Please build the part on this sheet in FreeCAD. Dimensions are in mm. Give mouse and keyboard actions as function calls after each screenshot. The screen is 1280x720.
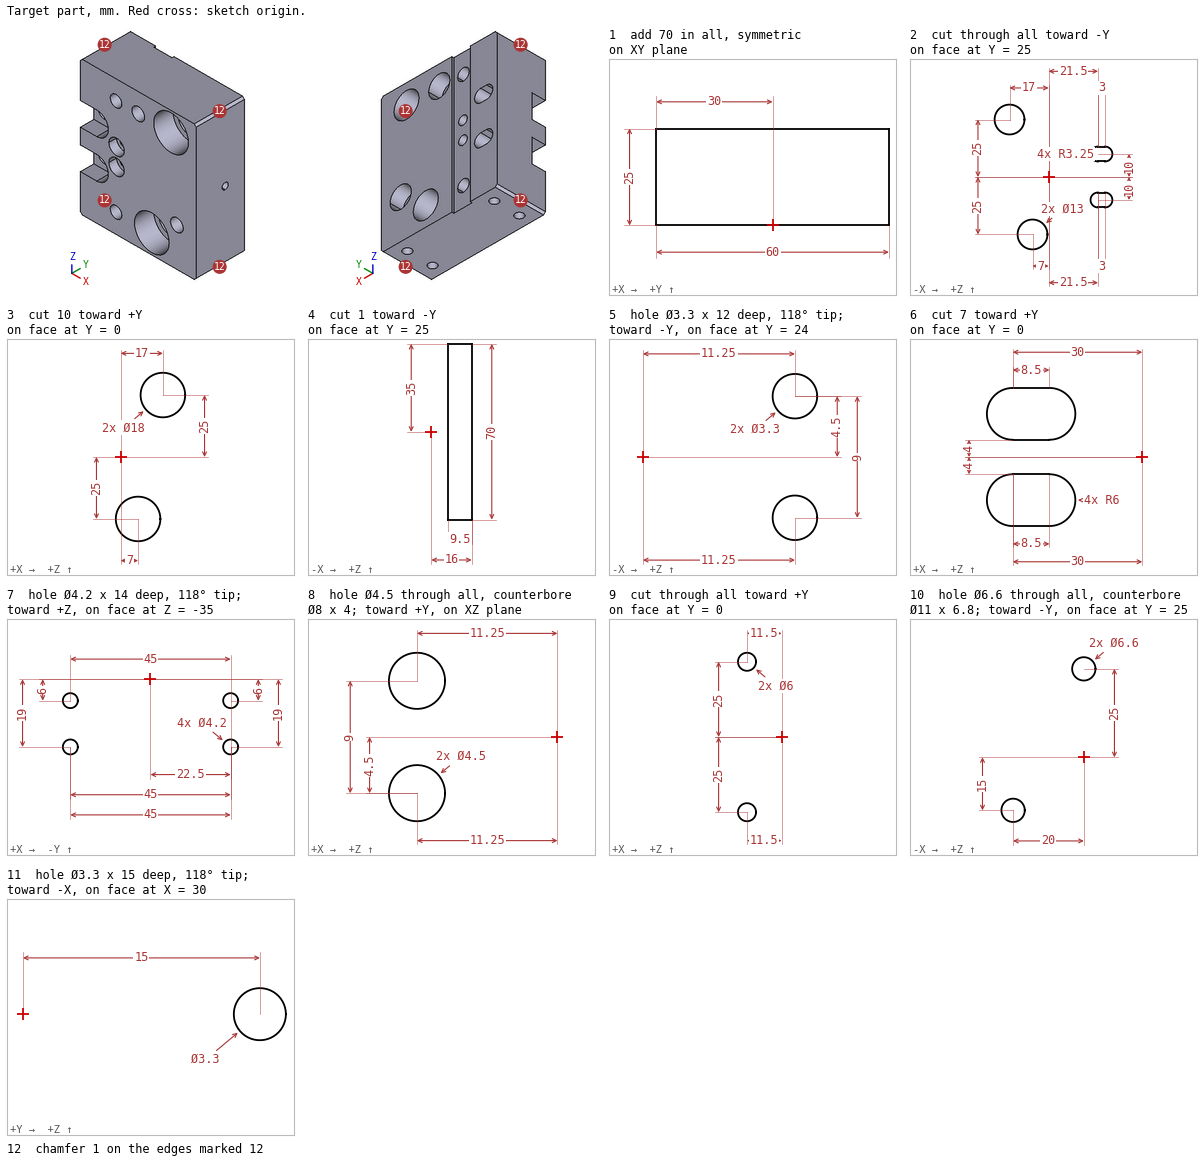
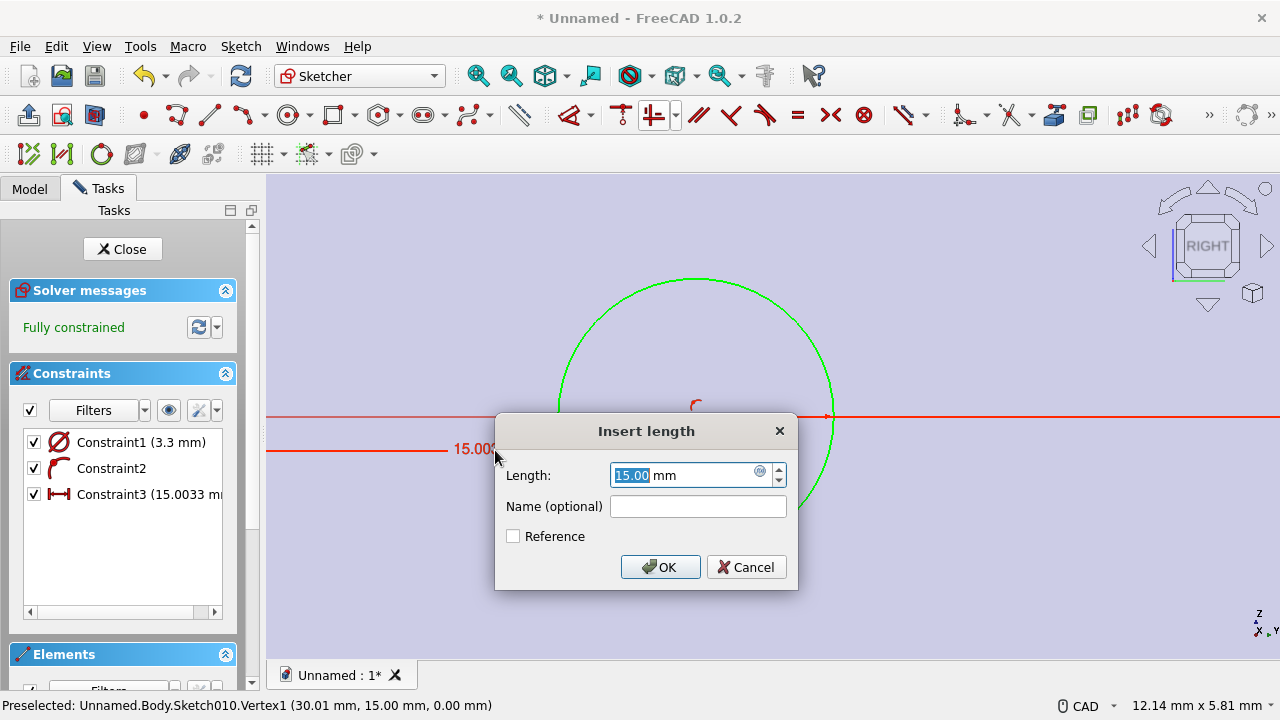
text(15)
key(Return)
key(Escape)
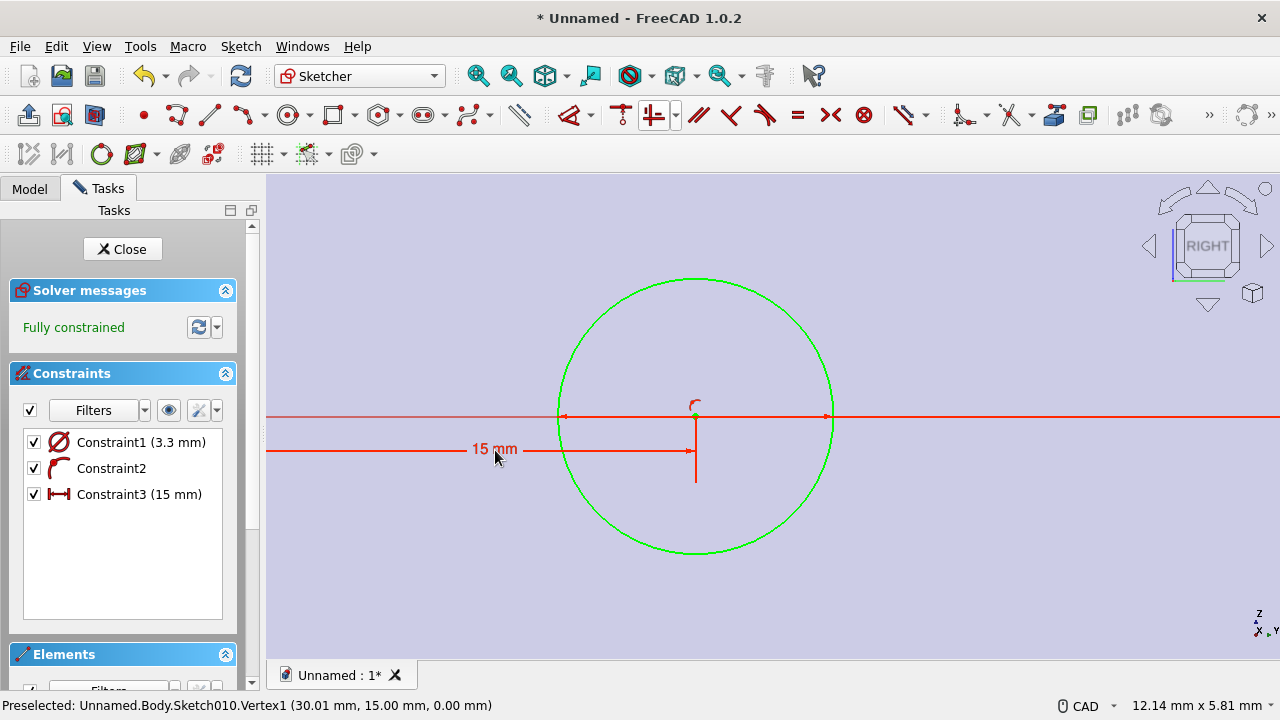
click(123, 249)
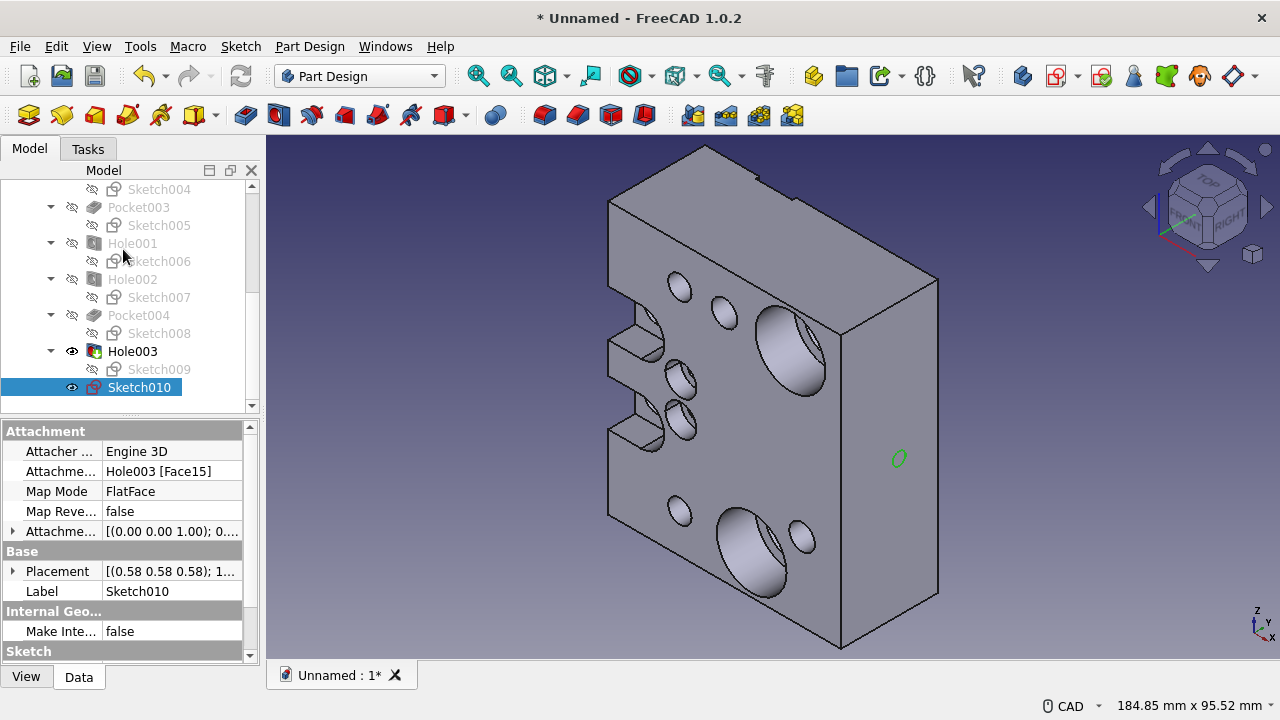
click(279, 116)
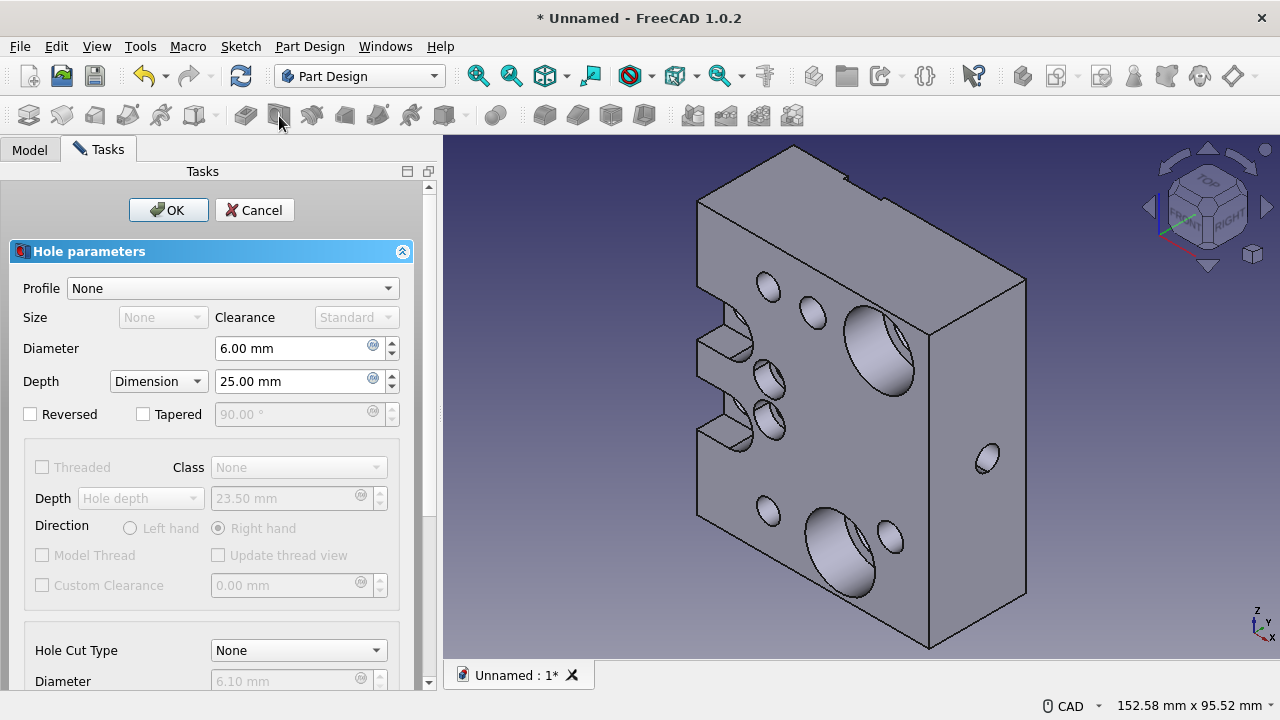
triple_click(300, 348)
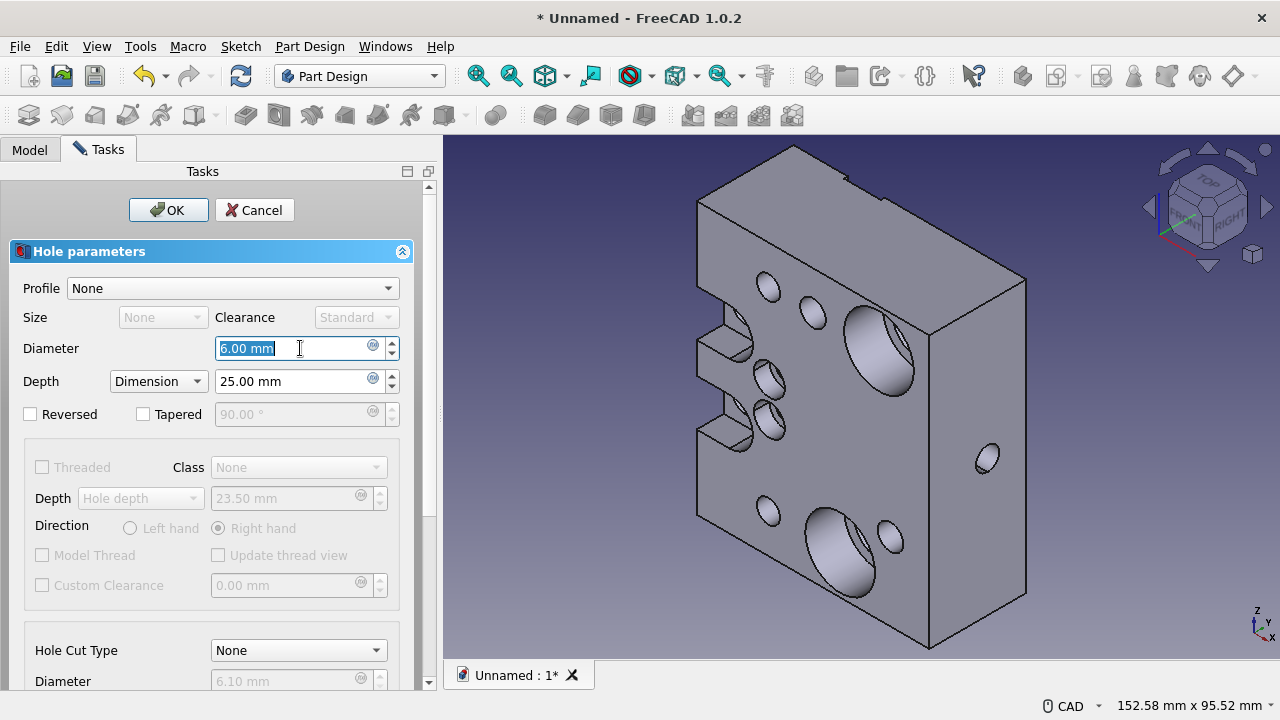
text(3.3)
key(Tab)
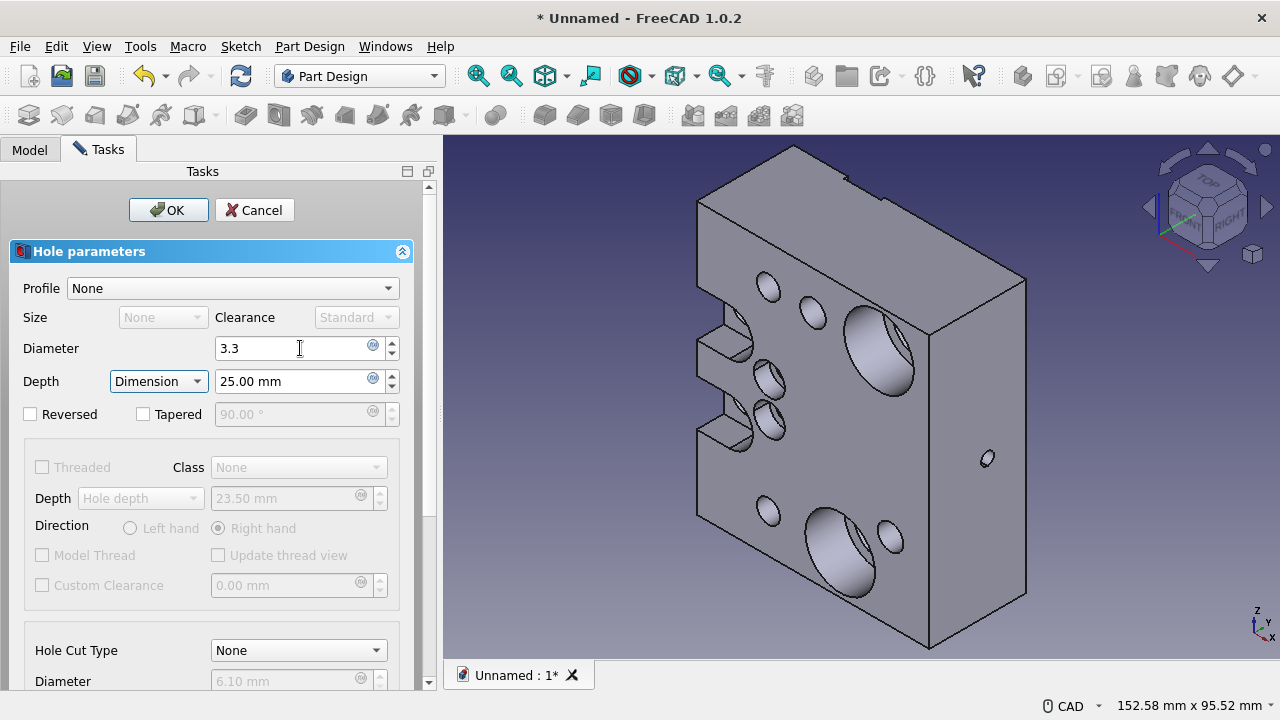
triple_click(300, 382)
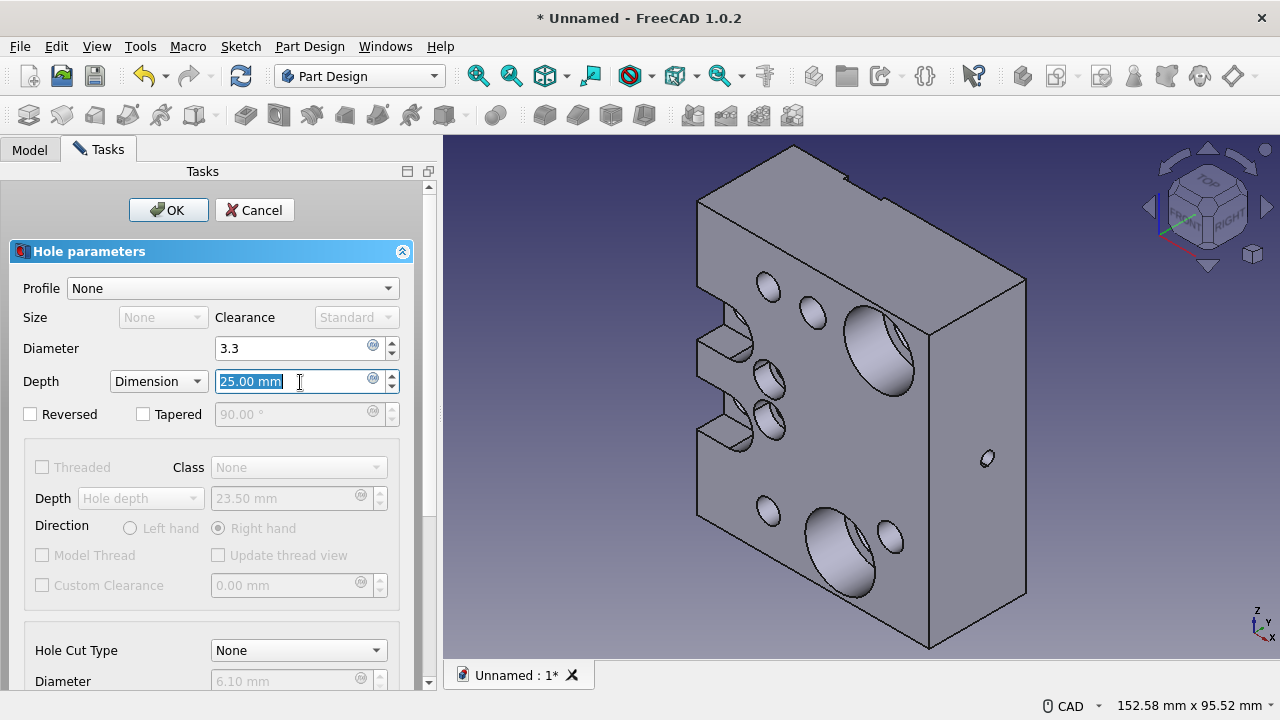
text(15)
key(Tab)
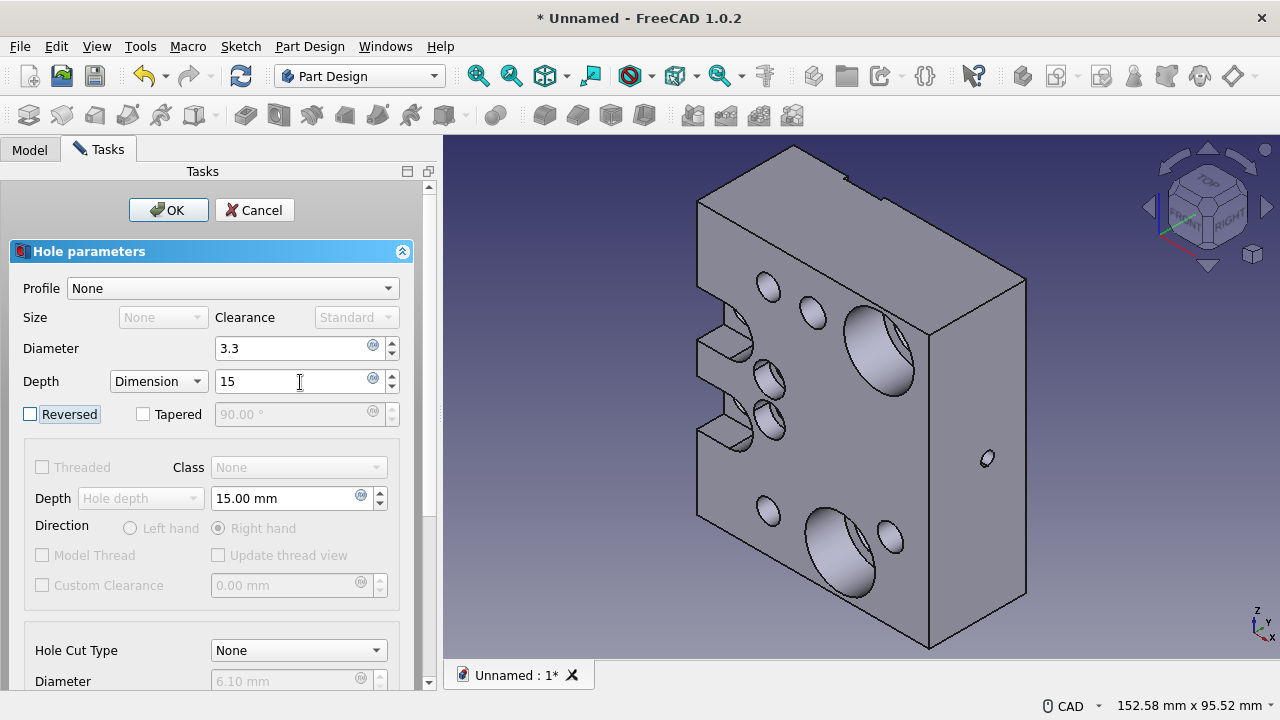
click(169, 210)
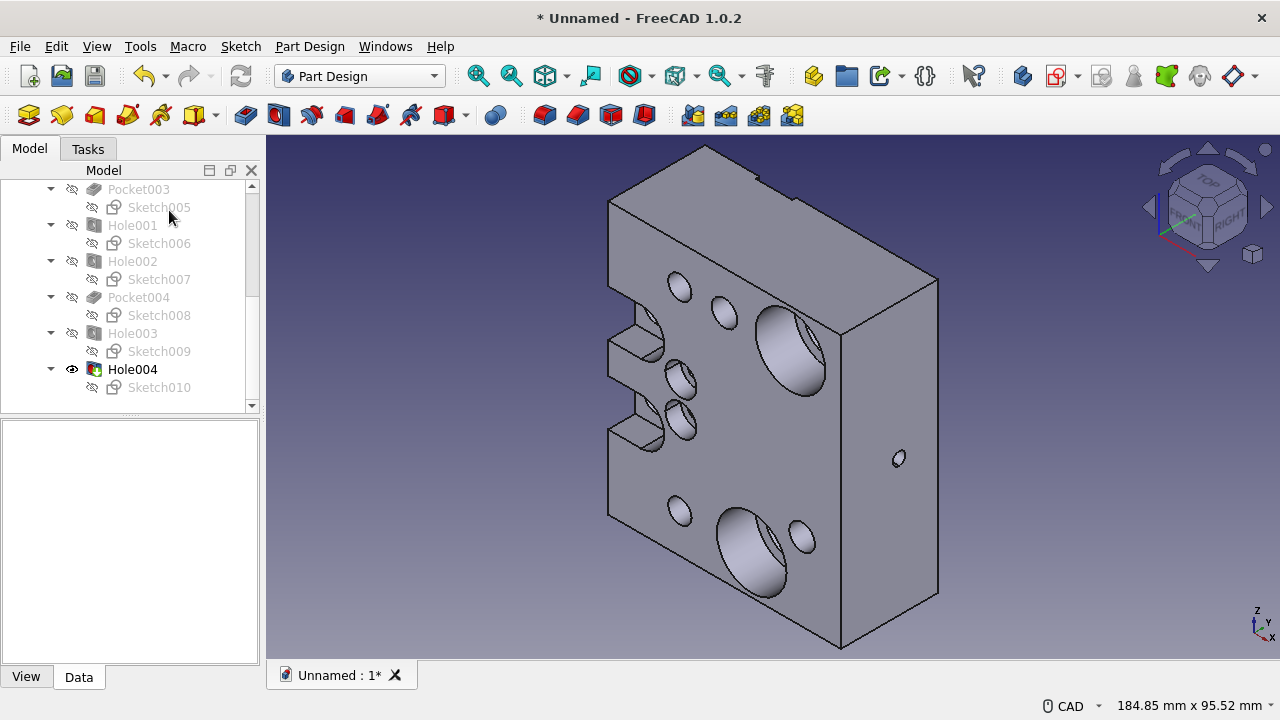
click(889, 306)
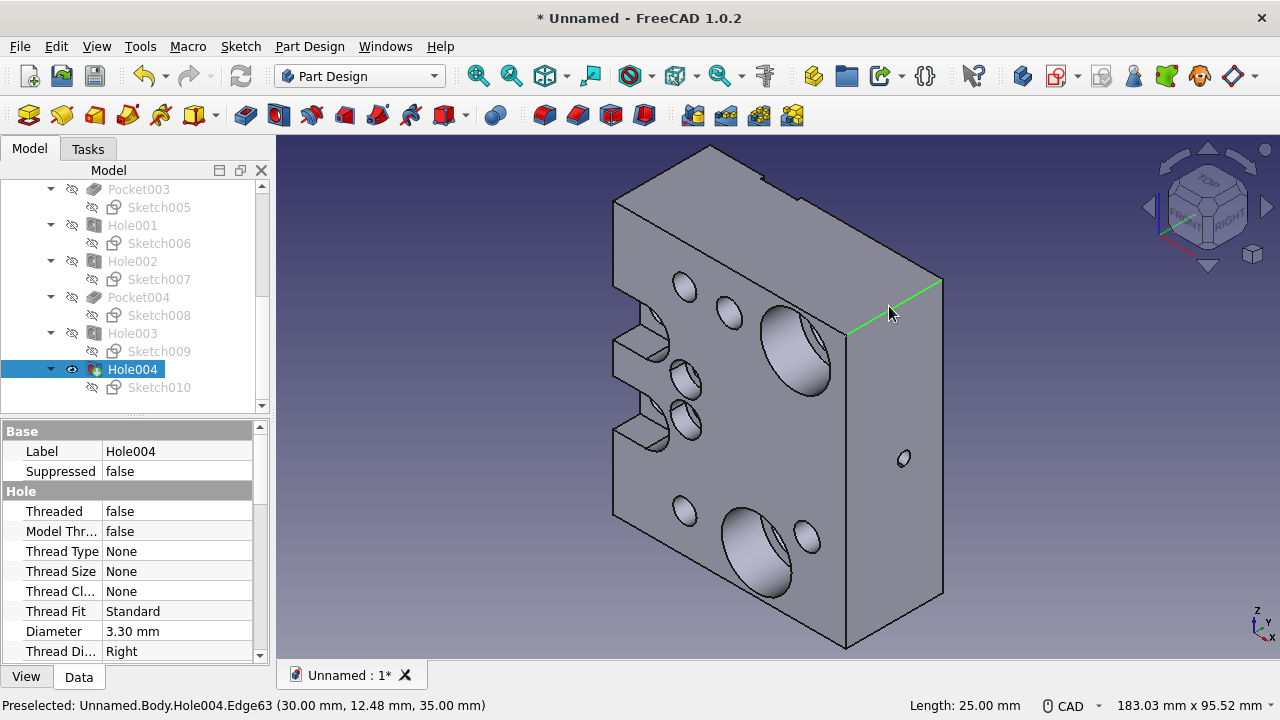
key(2)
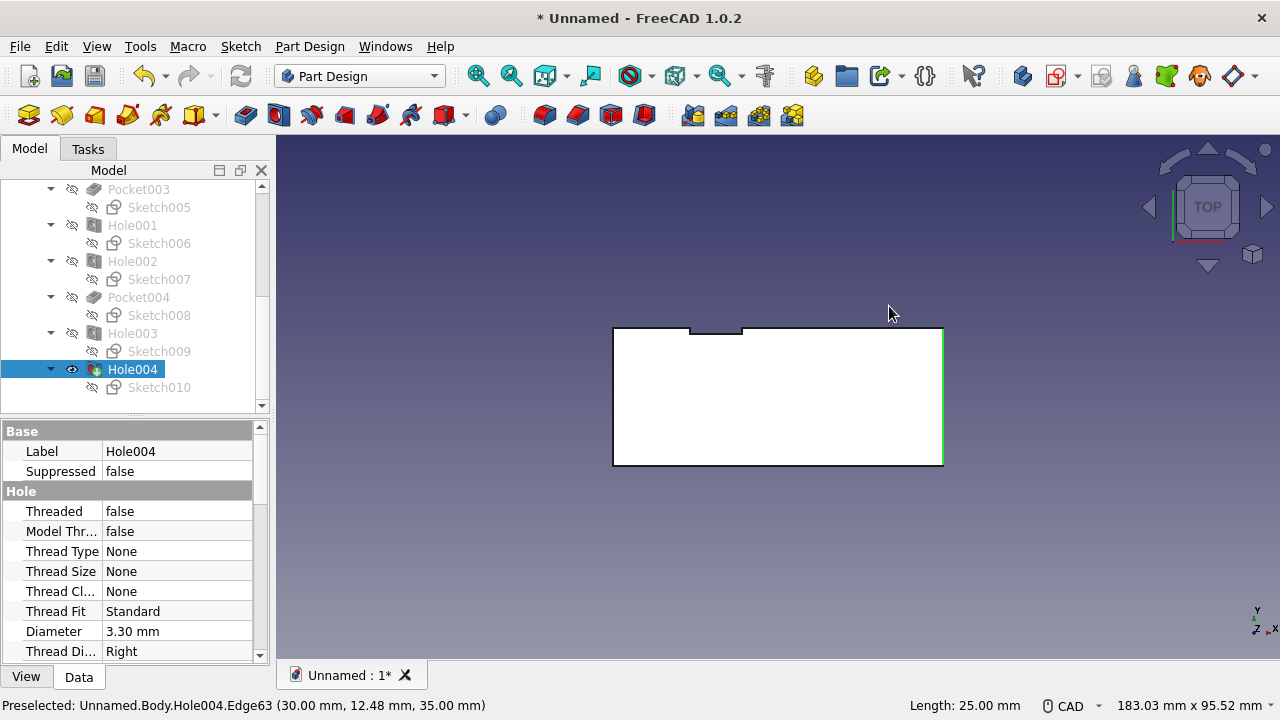
key(v)
key(f)